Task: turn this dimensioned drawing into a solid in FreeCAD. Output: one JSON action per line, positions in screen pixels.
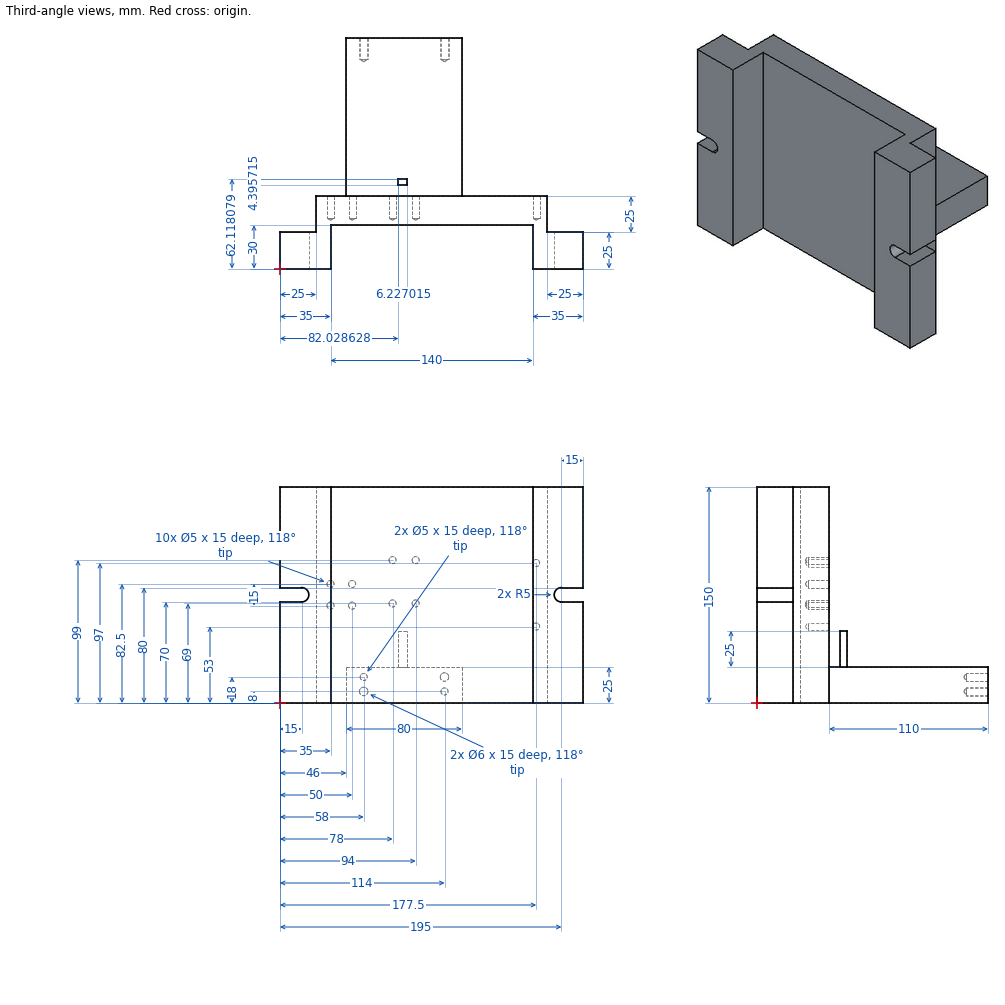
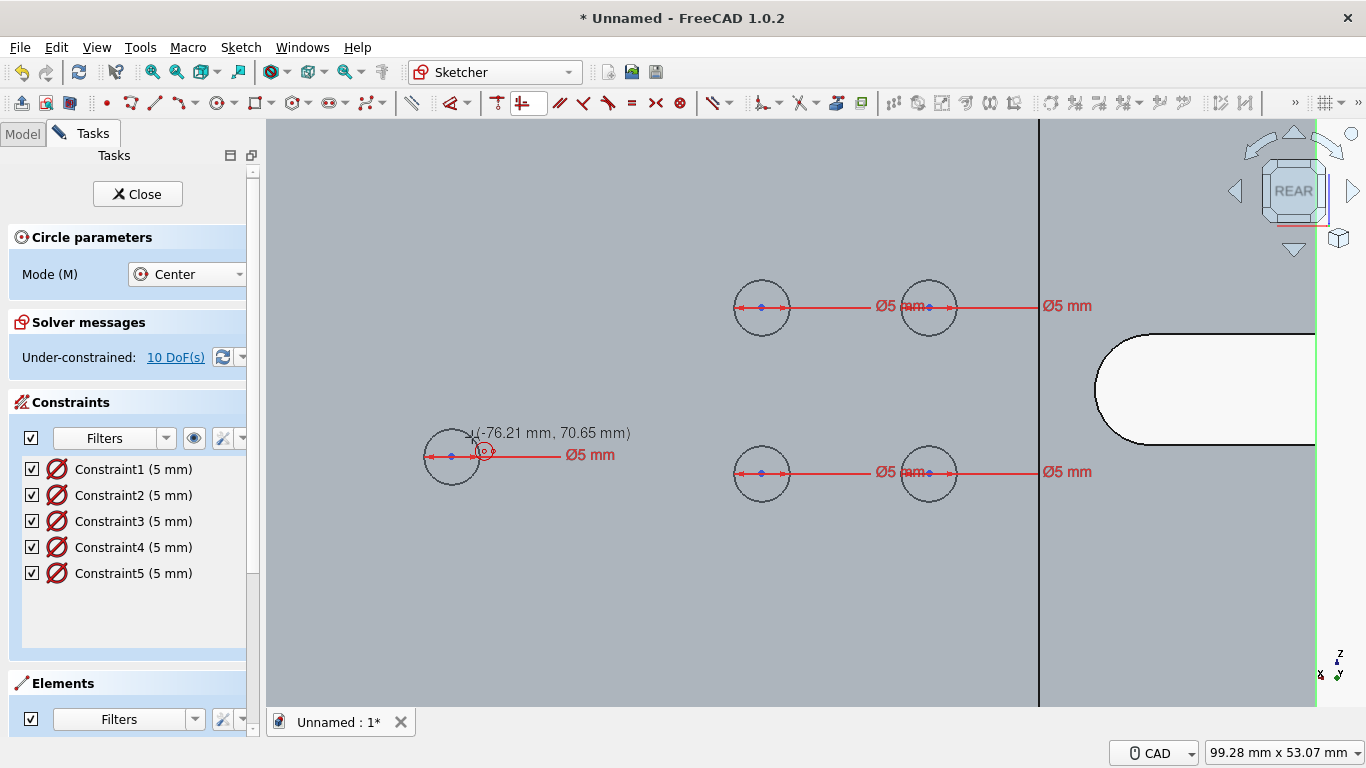
{"action": "scroll", "coordinate": [932, 307], "scroll_direction": "down", "scroll_amount": 6}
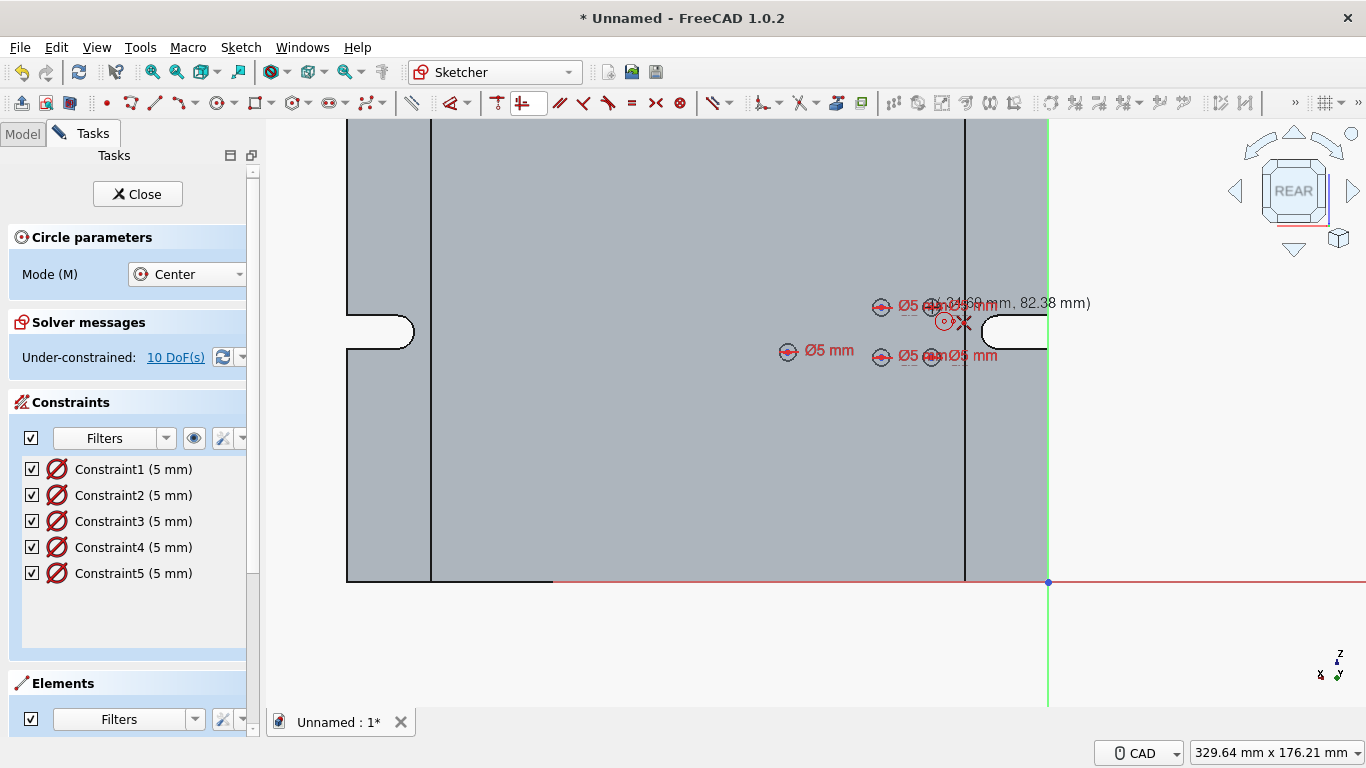
{"action": "scroll", "coordinate": [788, 252], "scroll_direction": "up", "scroll_amount": 6}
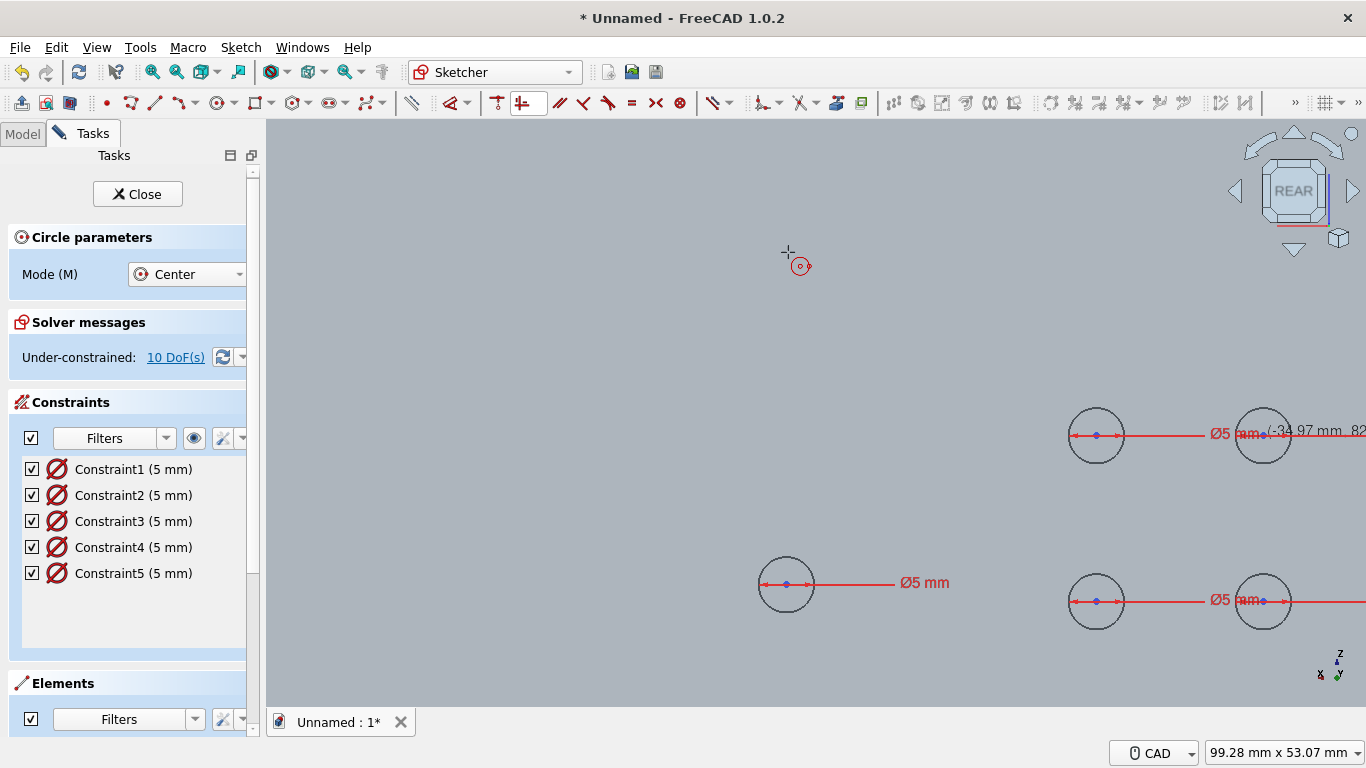
{"action": "left_click", "coordinate": [787, 252]}
{"action": "mouse_move", "coordinate": [806, 232]}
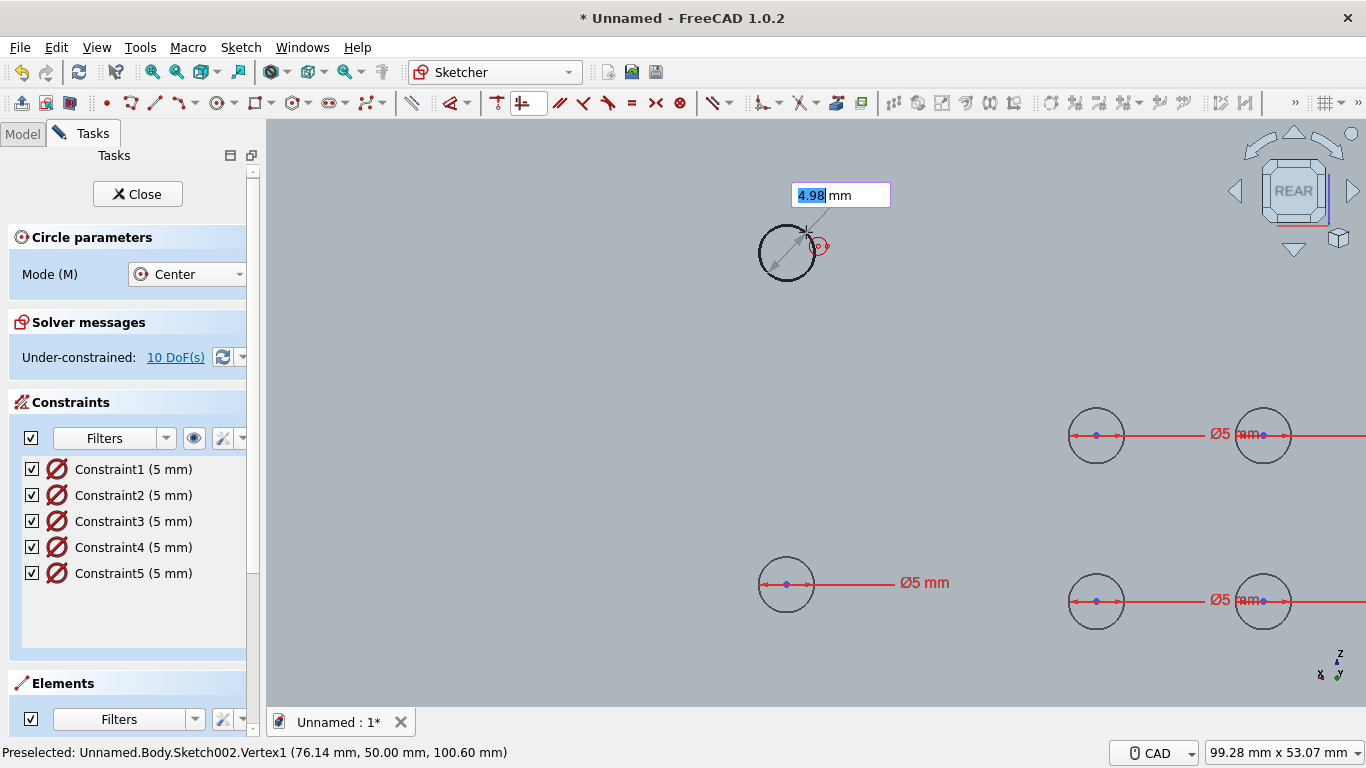
{"action": "type", "text": "5"}
{"action": "key", "text": "Return"}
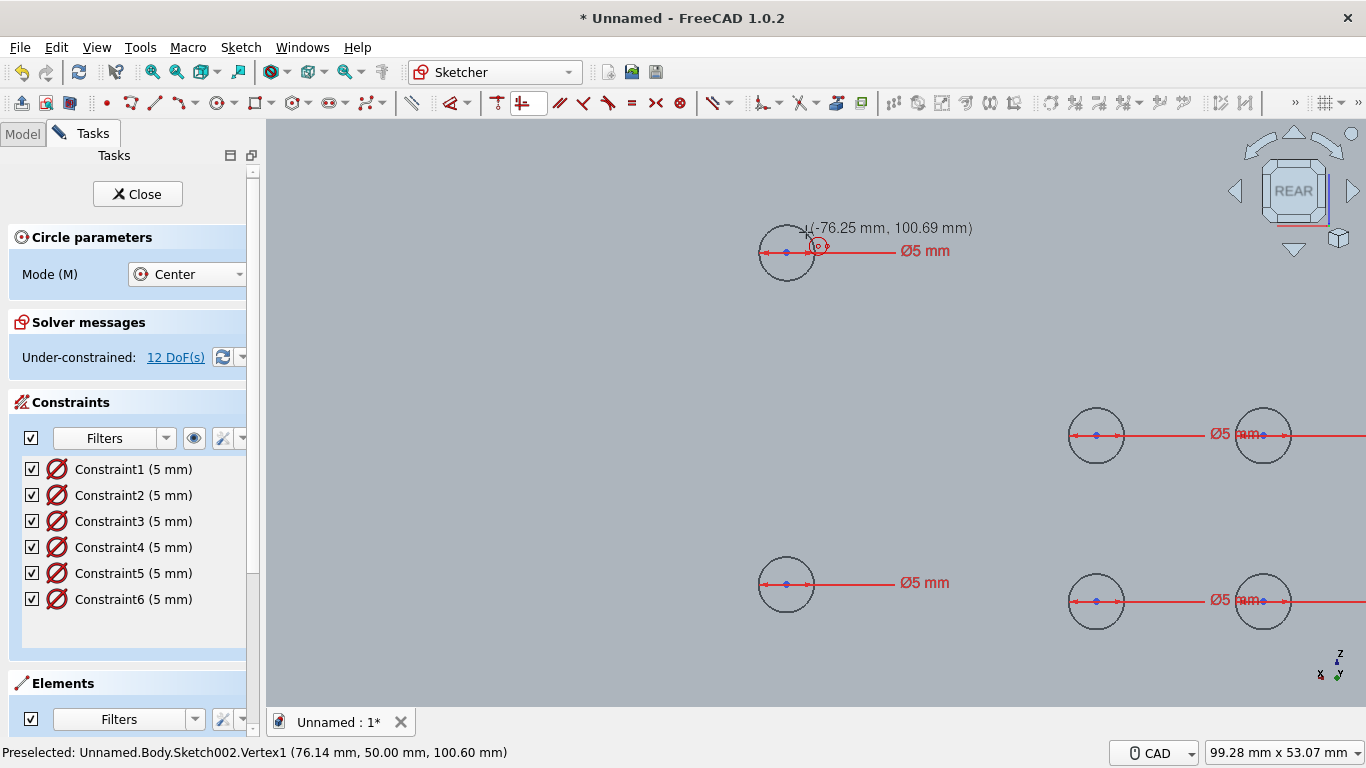
{"action": "left_click", "coordinate": [609, 584]}
{"action": "mouse_move", "coordinate": [629, 565]}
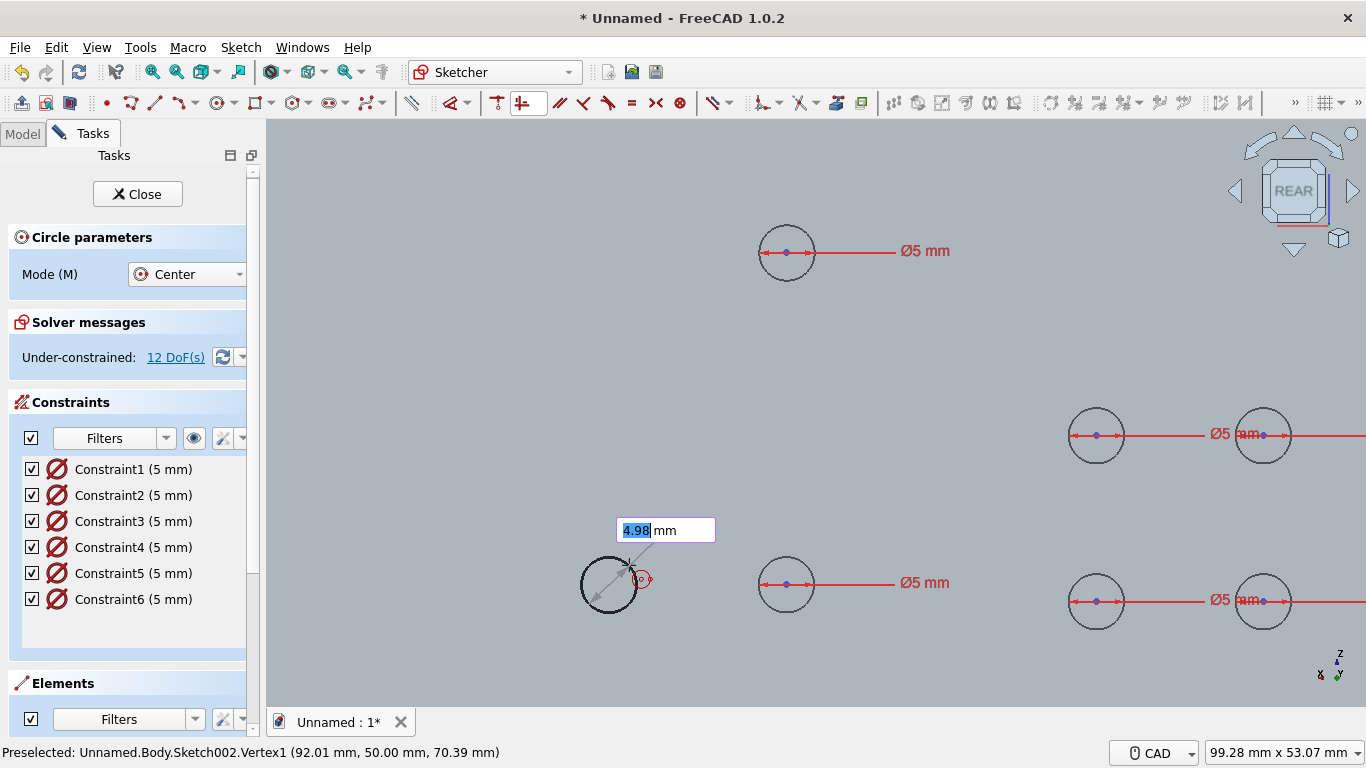
{"action": "type", "text": "5"}
{"action": "key", "text": "Return"}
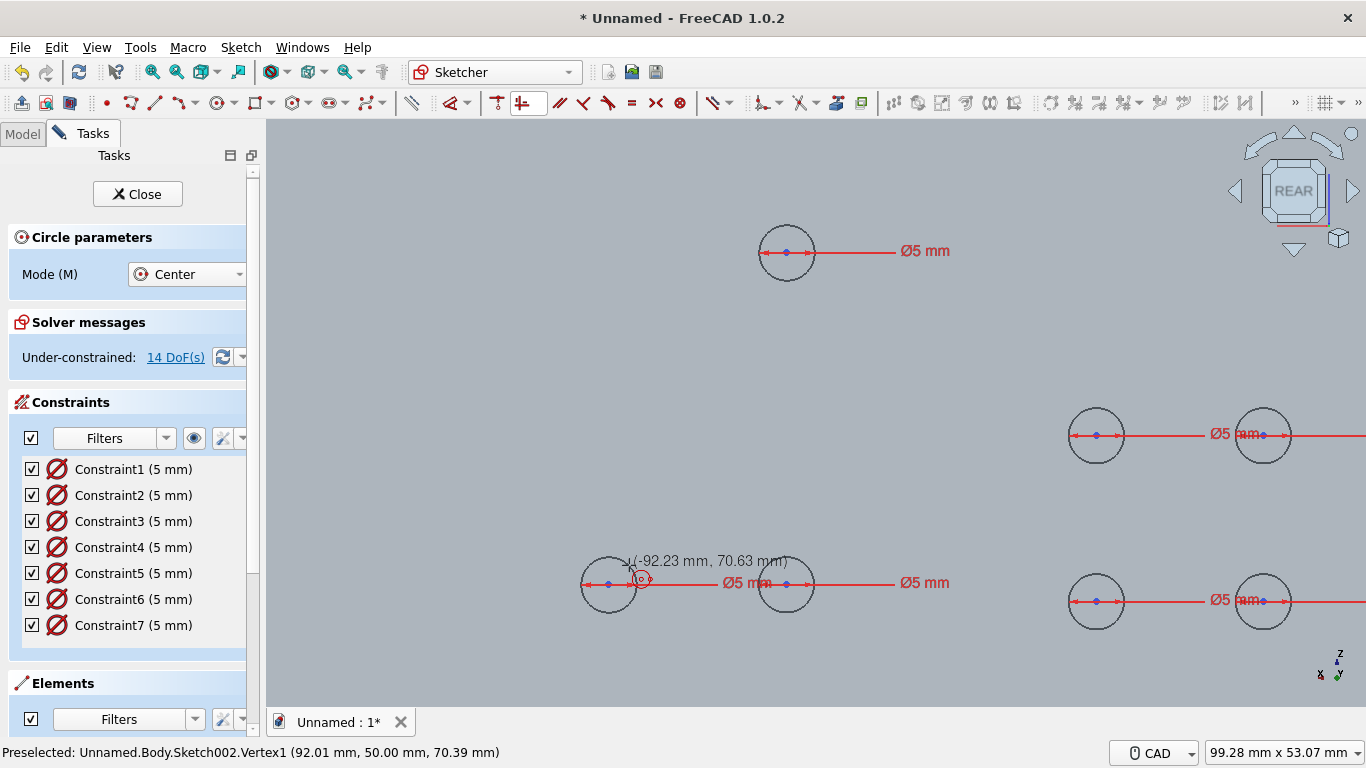
{"action": "left_click", "coordinate": [609, 252]}
{"action": "mouse_move", "coordinate": [629, 232]}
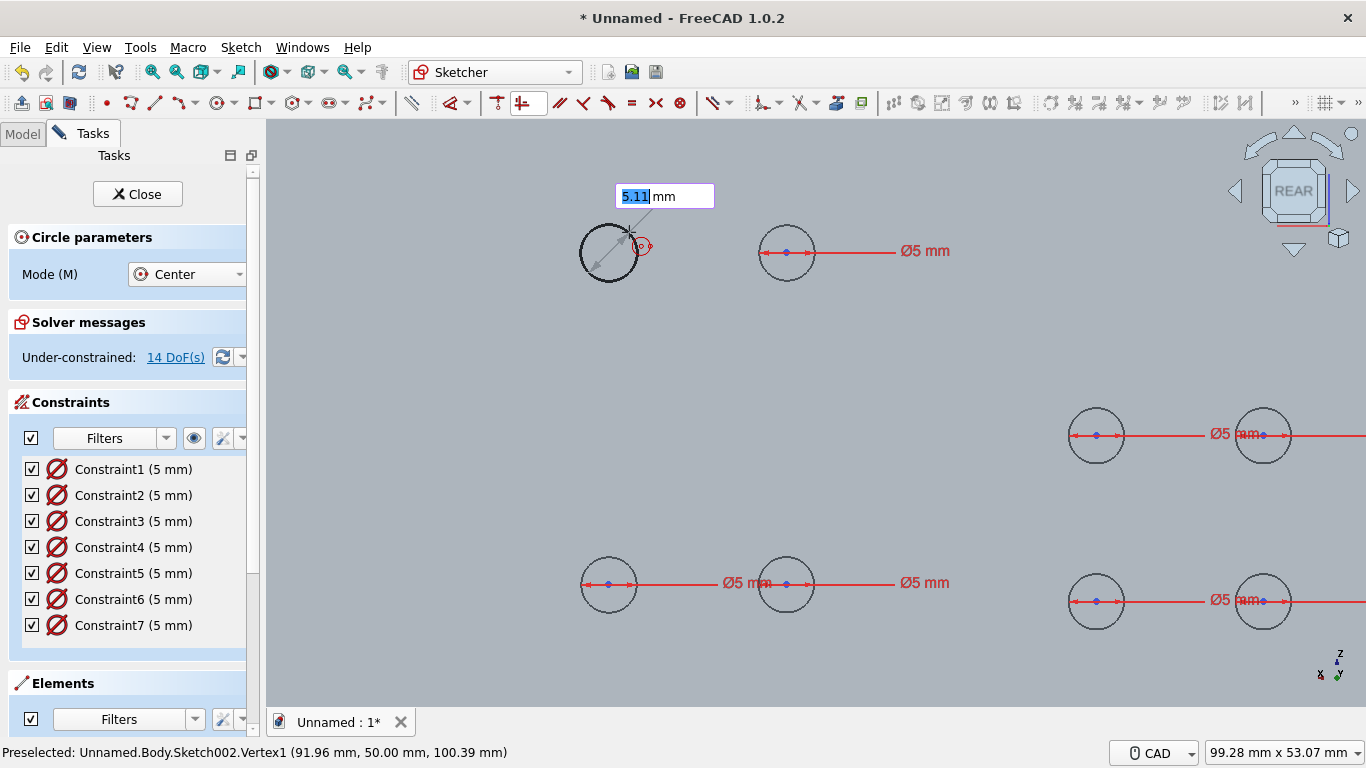
{"action": "type", "text": "5"}
{"action": "key", "text": "Return"}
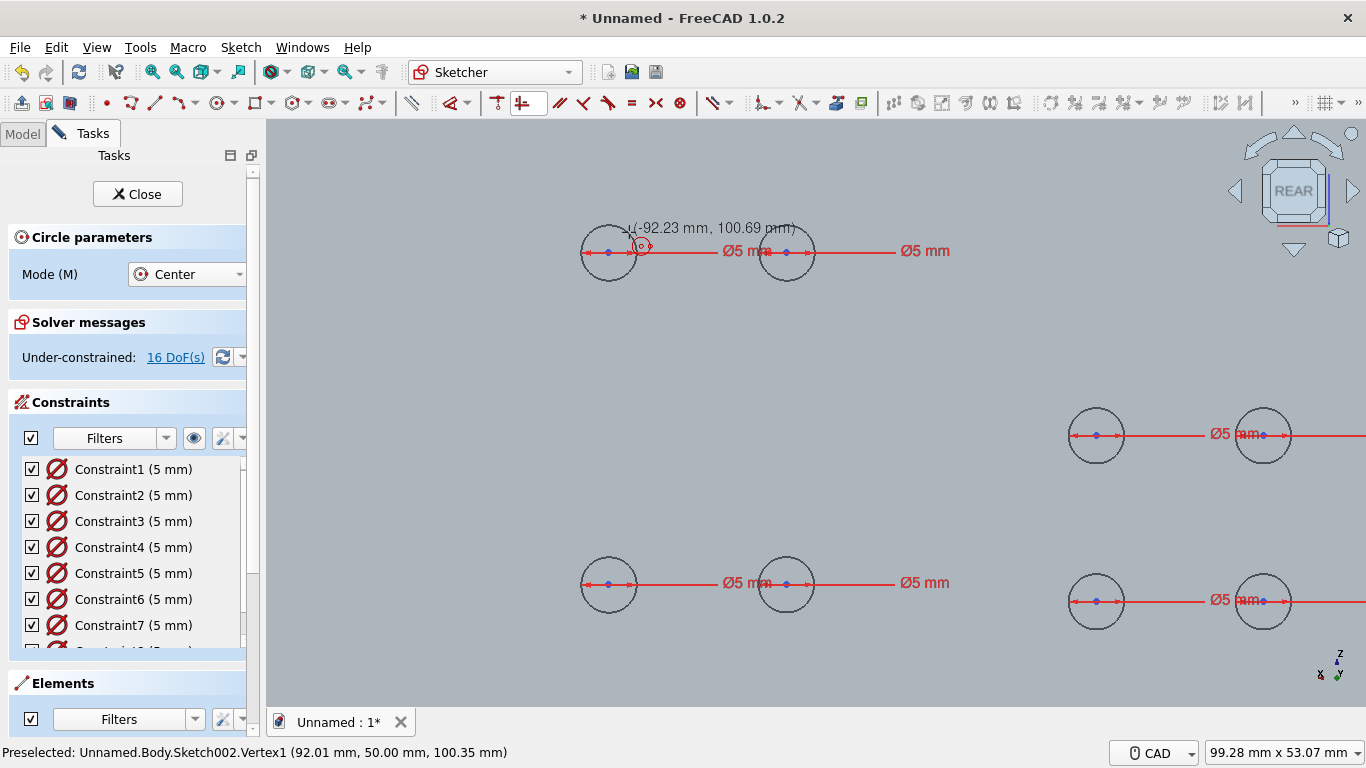
{"action": "scroll", "coordinate": [788, 252], "scroll_direction": "down", "scroll_amount": 6}